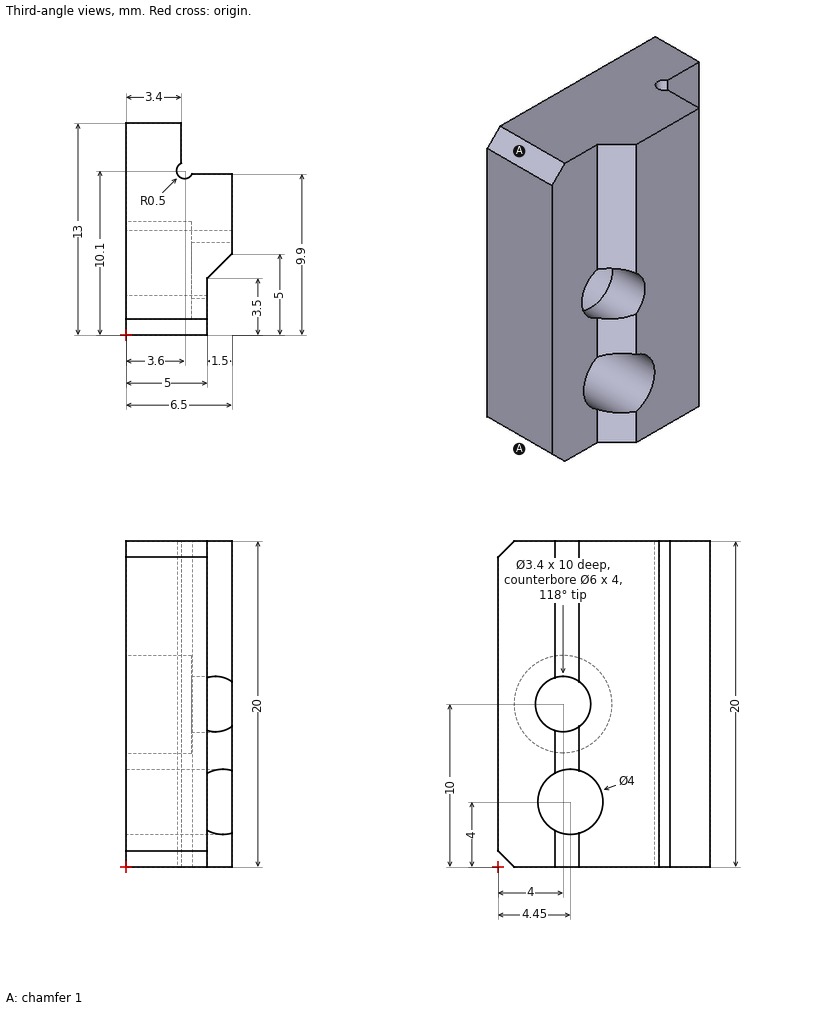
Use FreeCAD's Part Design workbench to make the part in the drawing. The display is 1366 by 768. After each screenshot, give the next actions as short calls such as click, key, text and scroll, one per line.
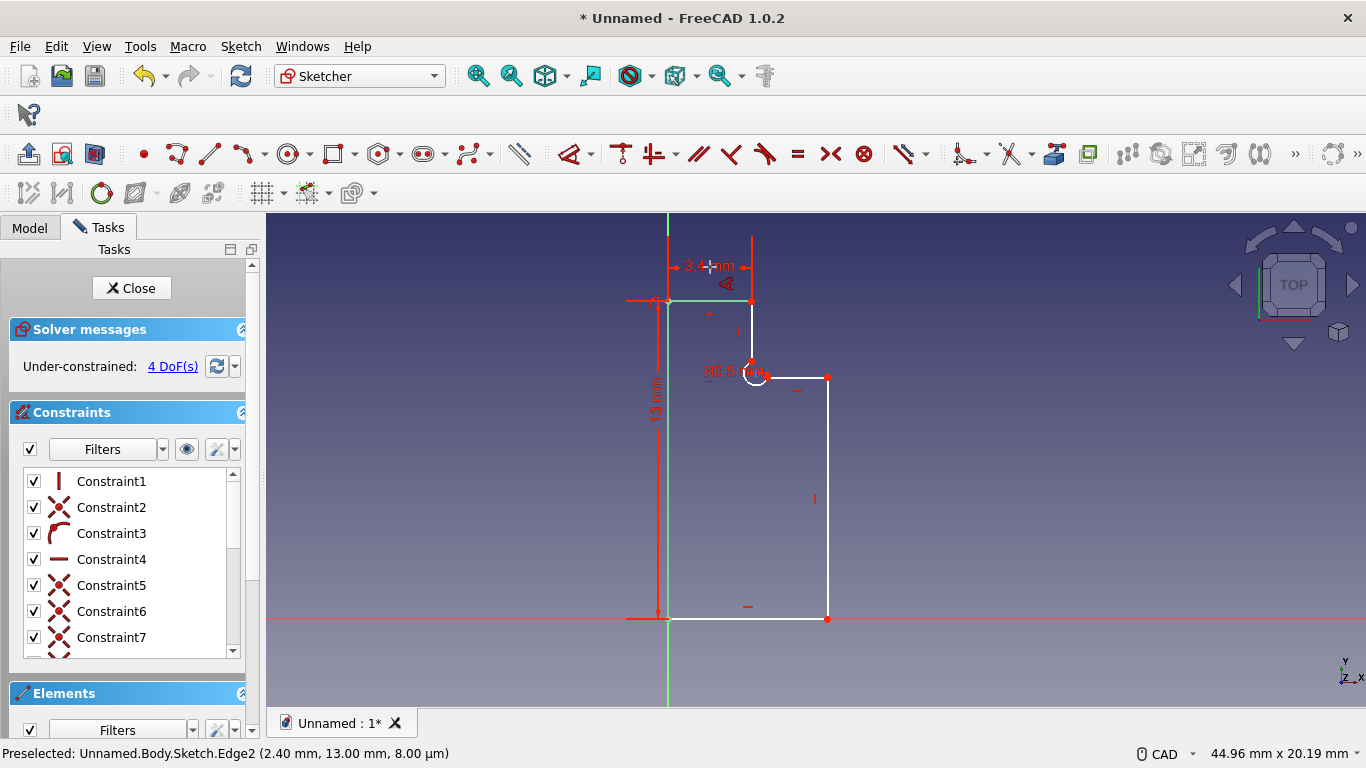
click(716, 619)
click(748, 653)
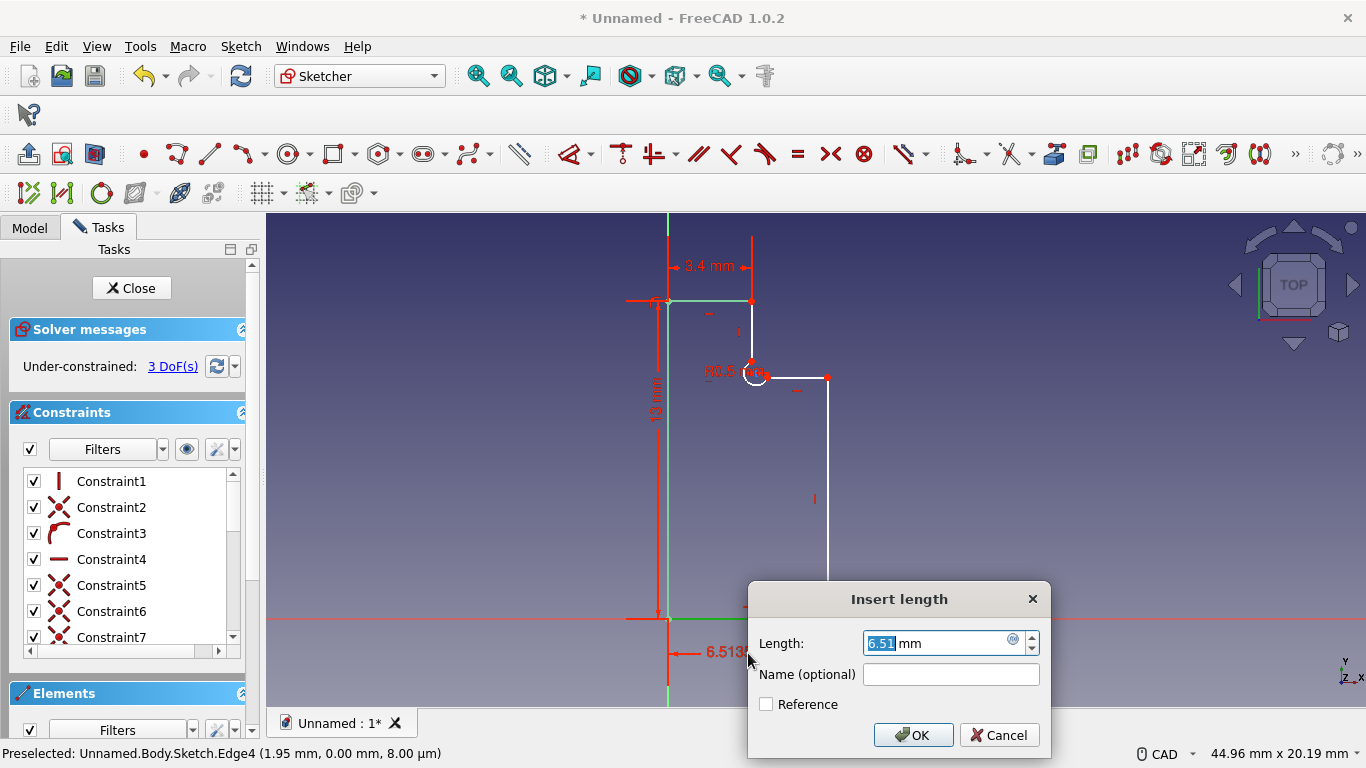
text(6.5)
key(Return)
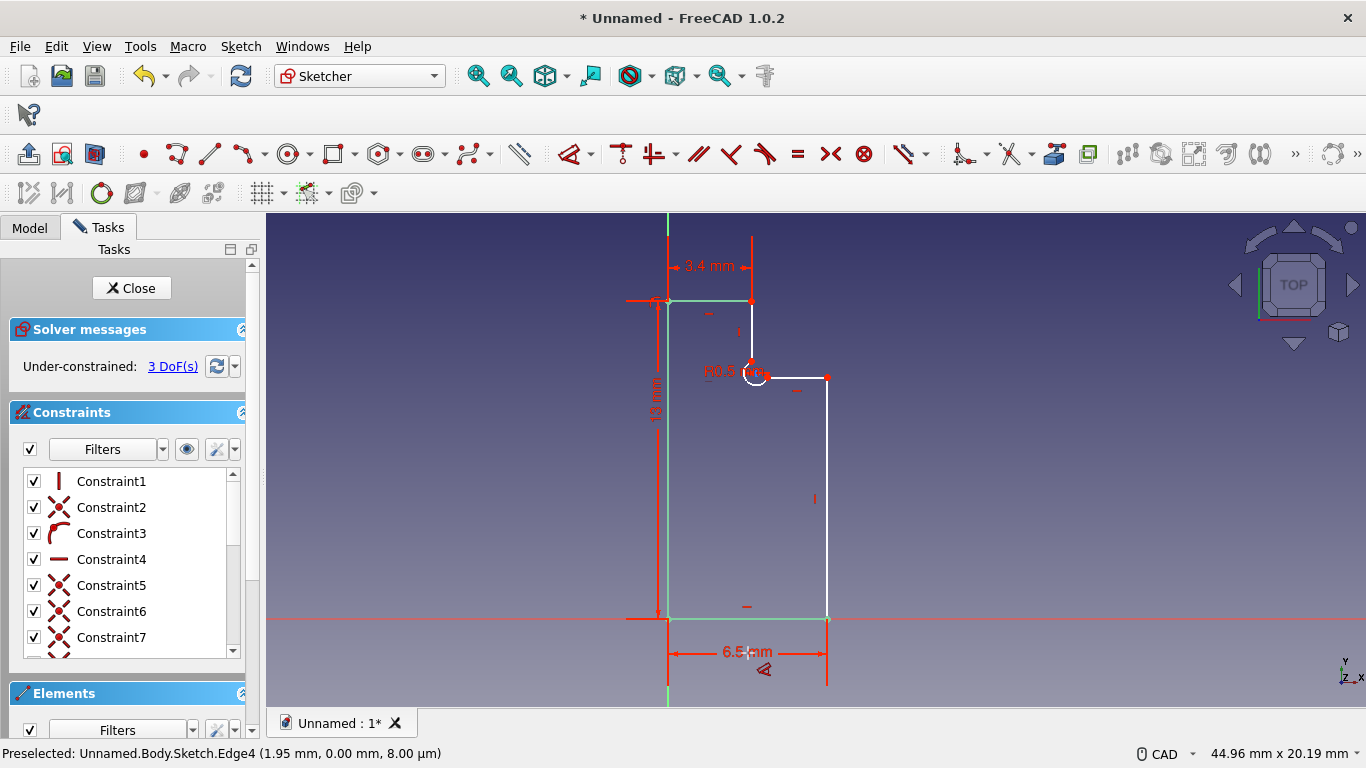
click(827, 547)
click(861, 499)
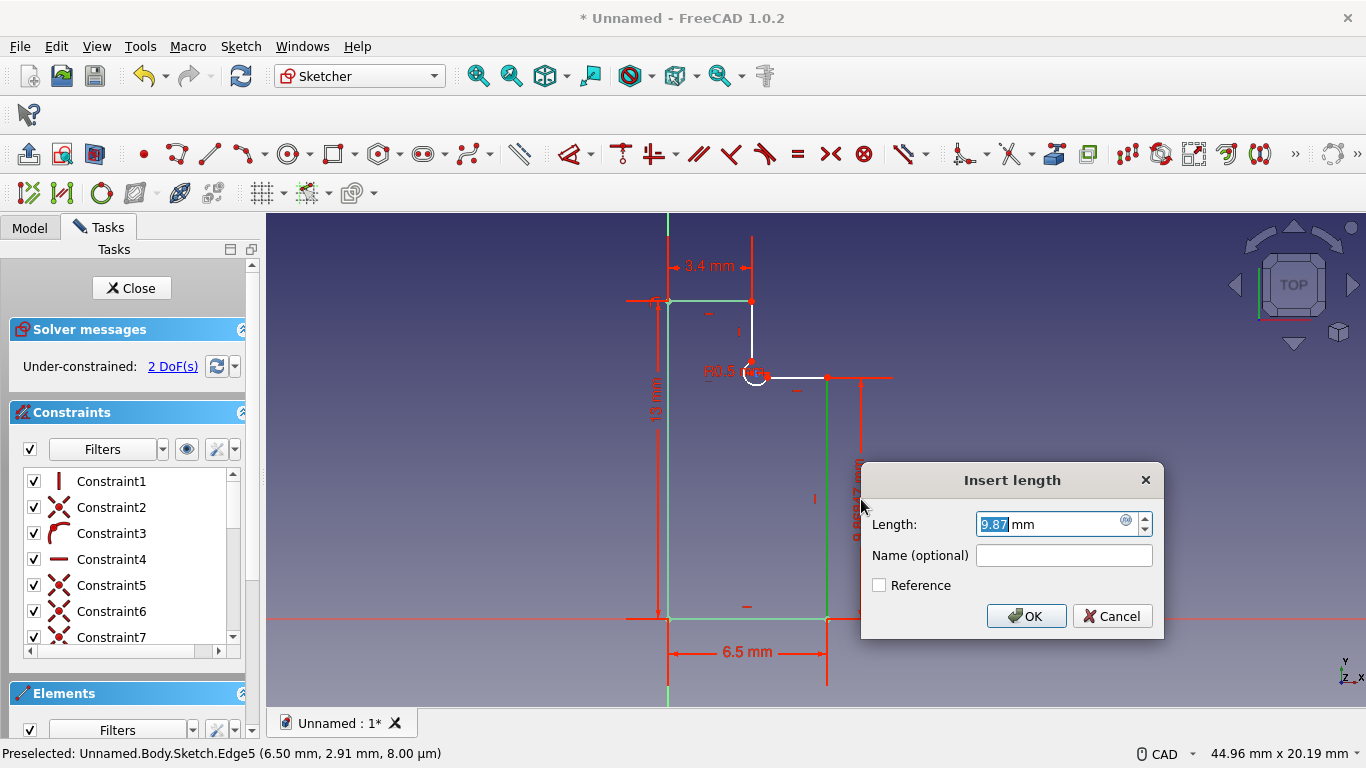
text(9.9)
key(Return)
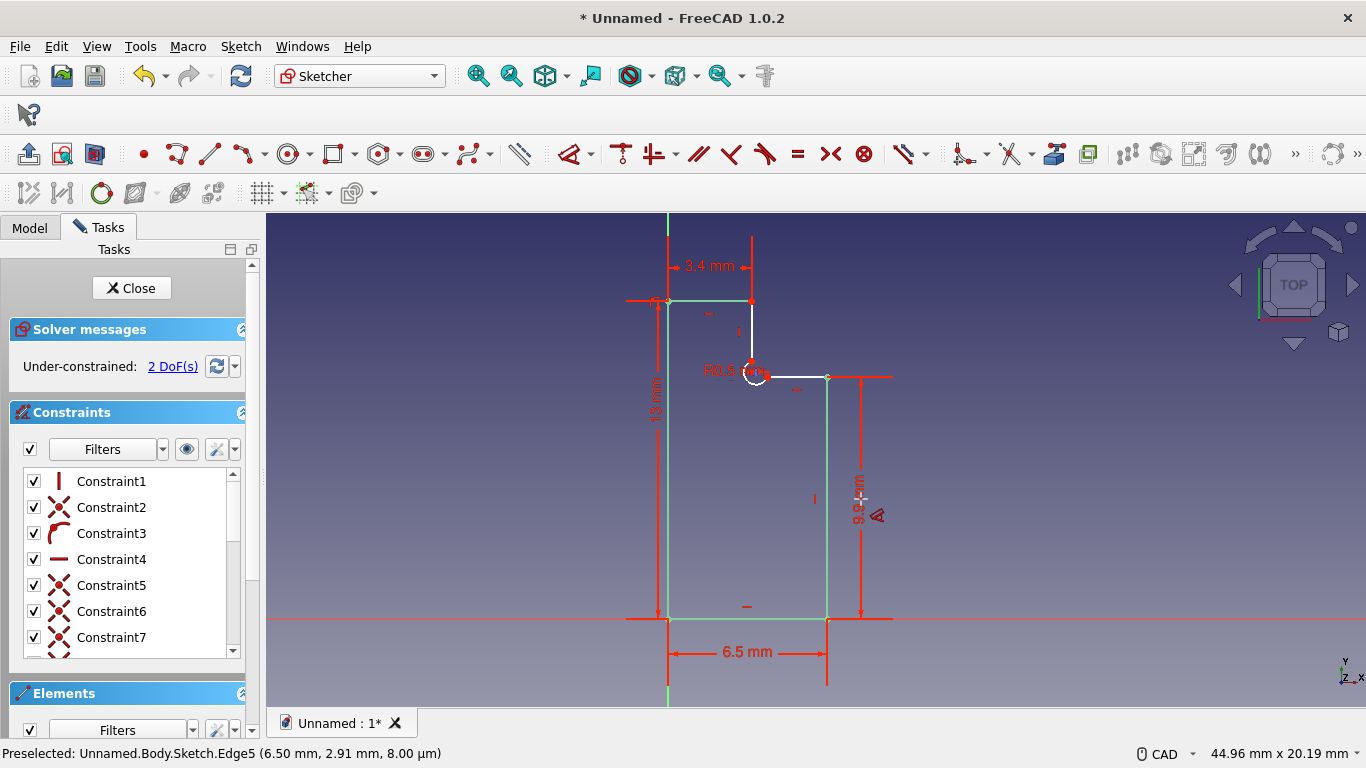
click(756, 372)
click(712, 338)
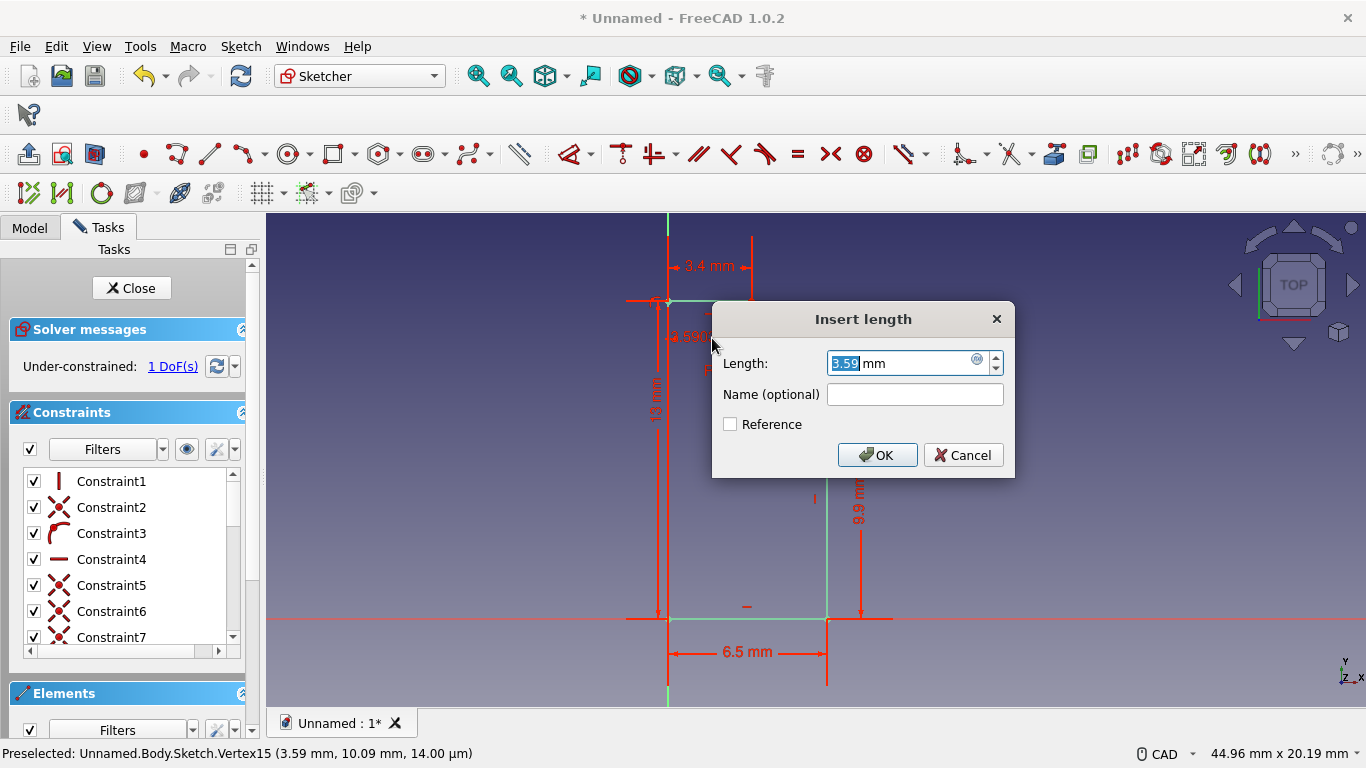
text(3.6)
key(Return)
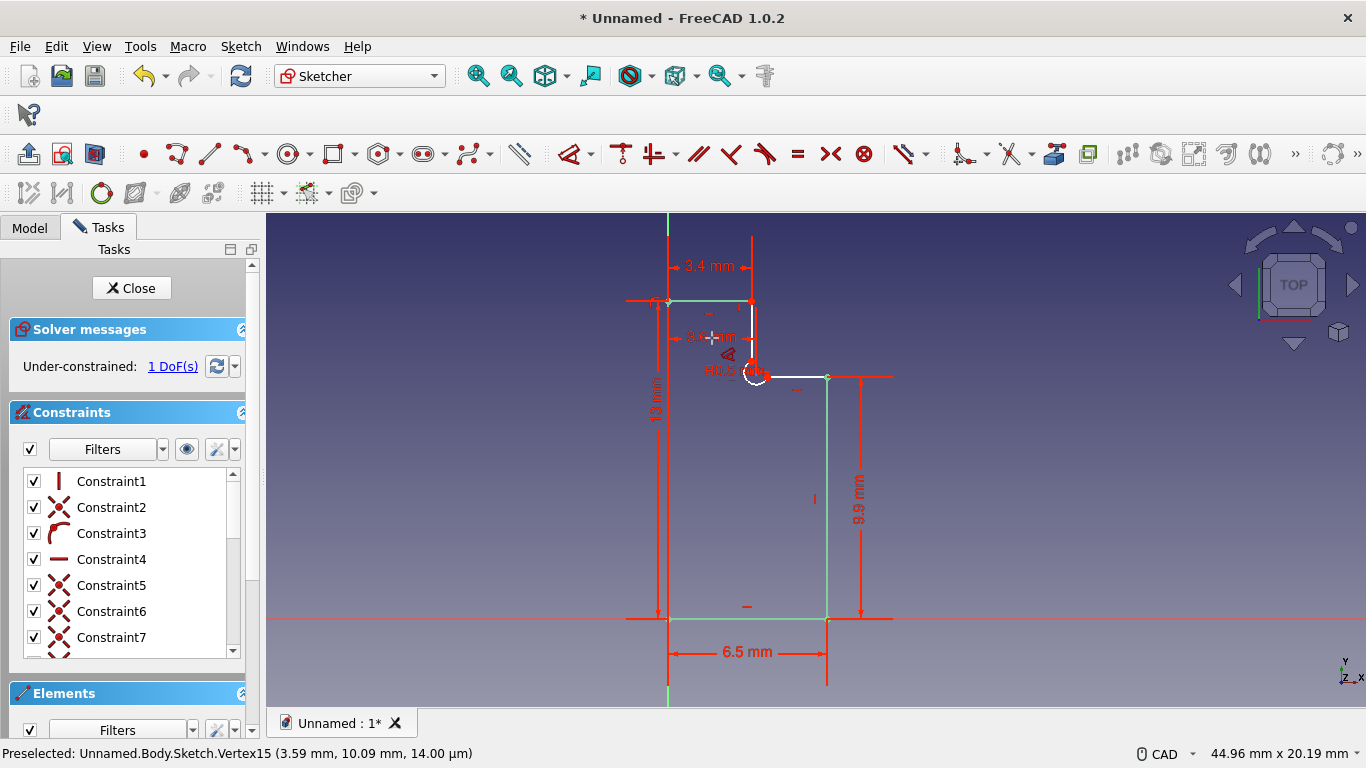
click(756, 372)
click(634, 496)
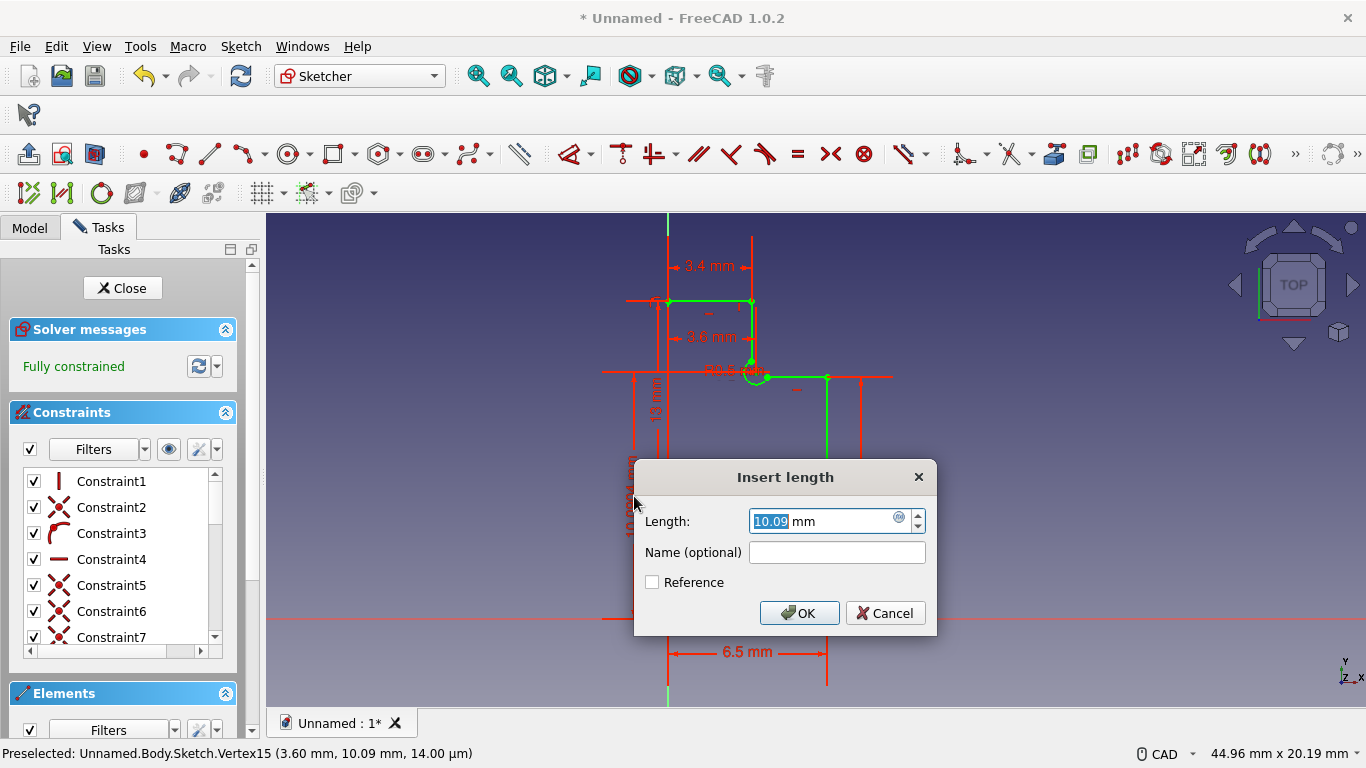
text(10.1)
key(Return)
key(Escape)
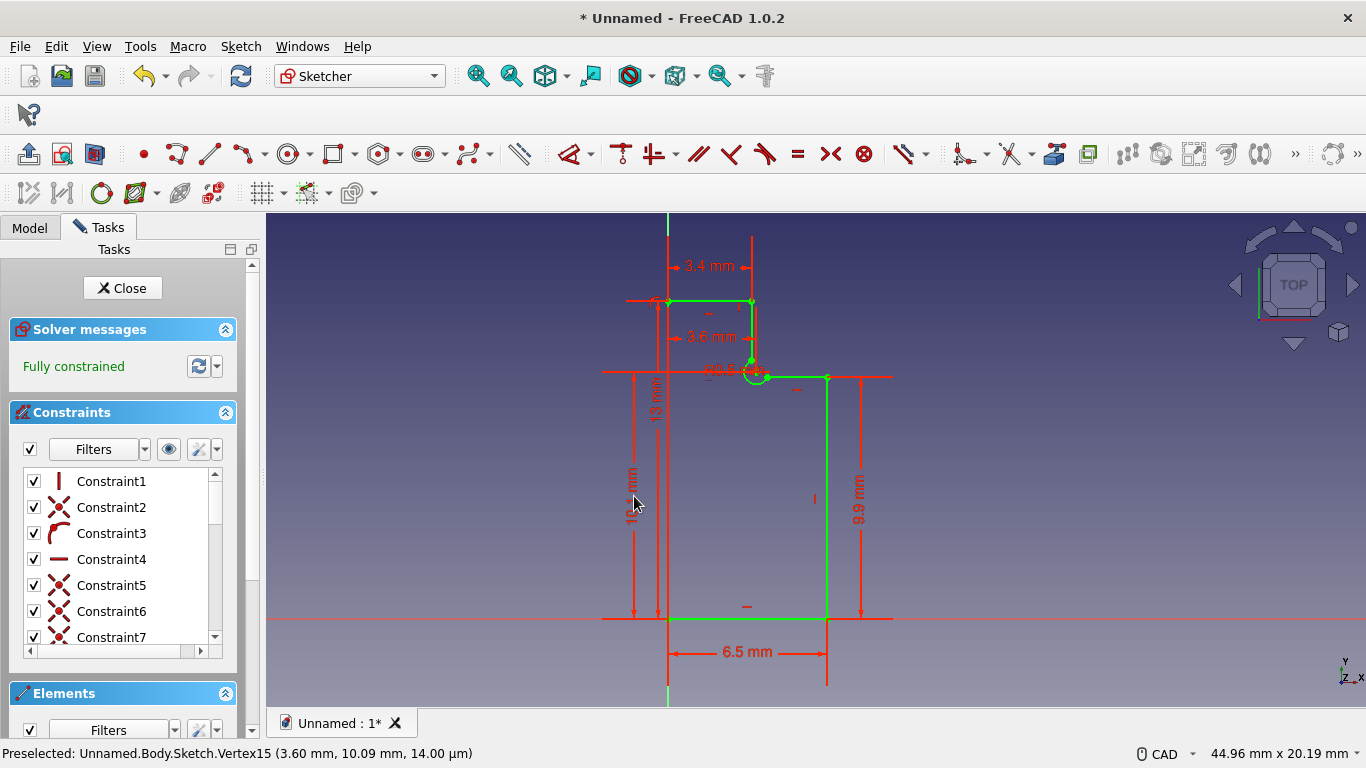
click(123, 288)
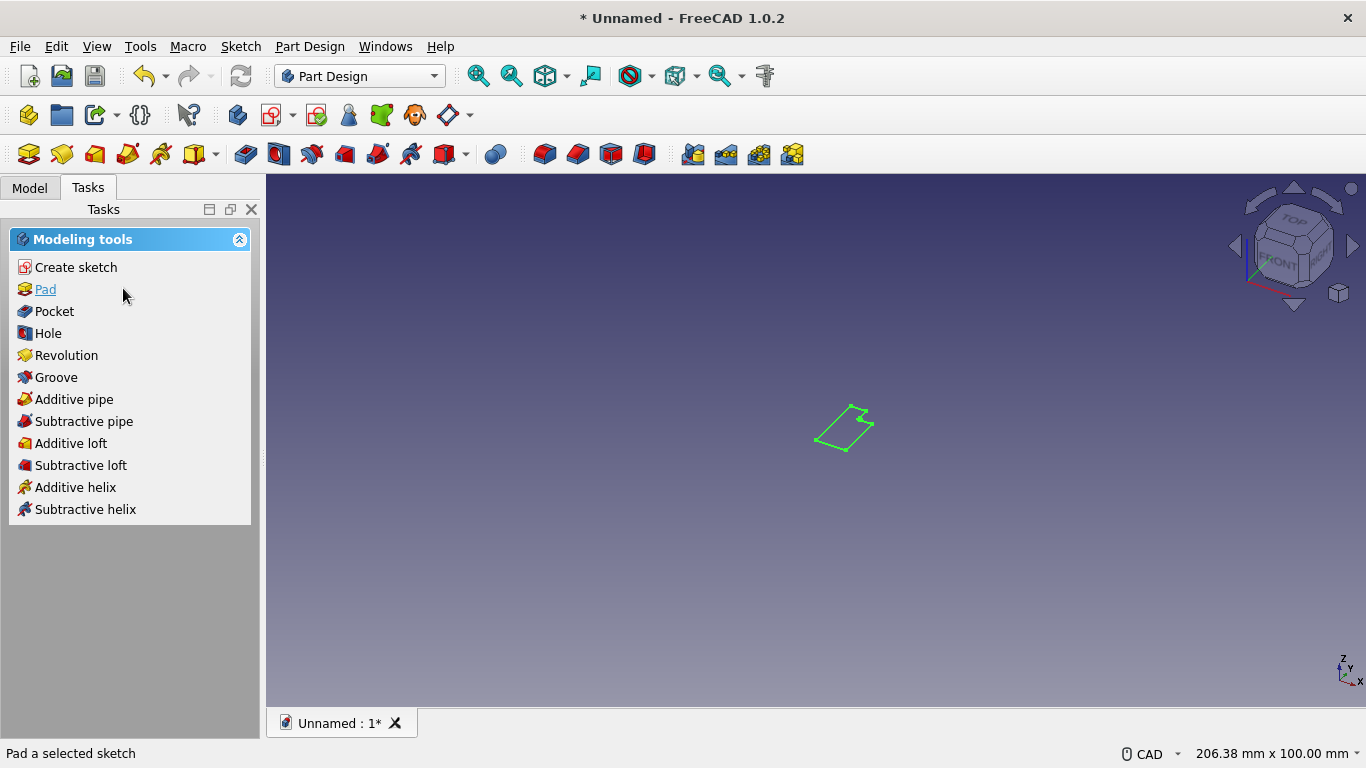
click(29, 154)